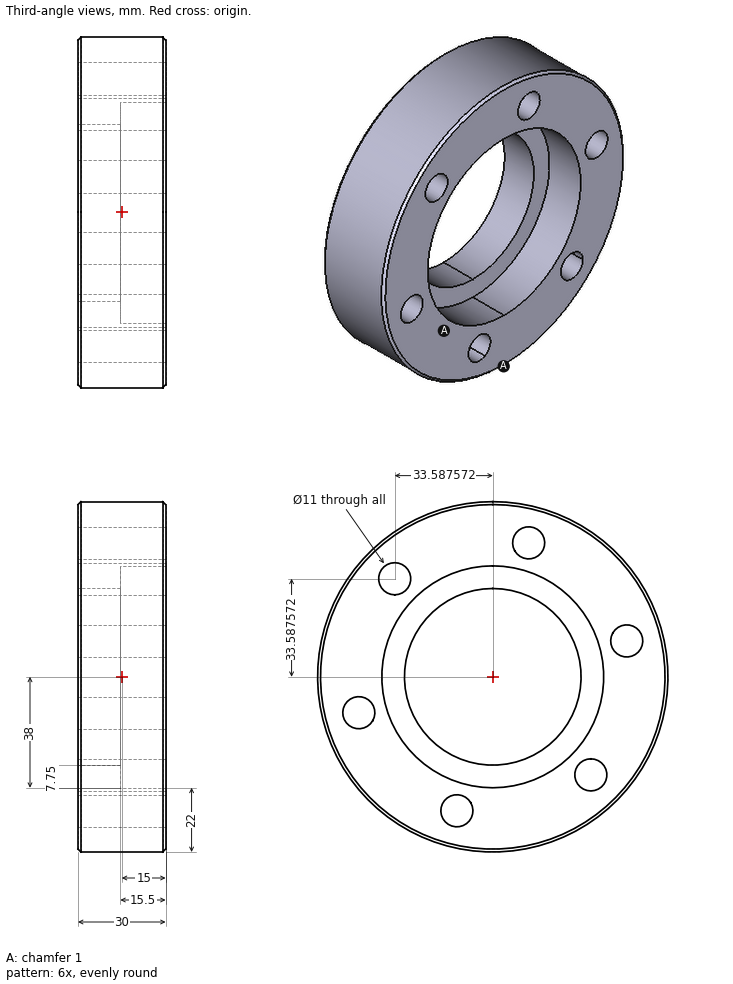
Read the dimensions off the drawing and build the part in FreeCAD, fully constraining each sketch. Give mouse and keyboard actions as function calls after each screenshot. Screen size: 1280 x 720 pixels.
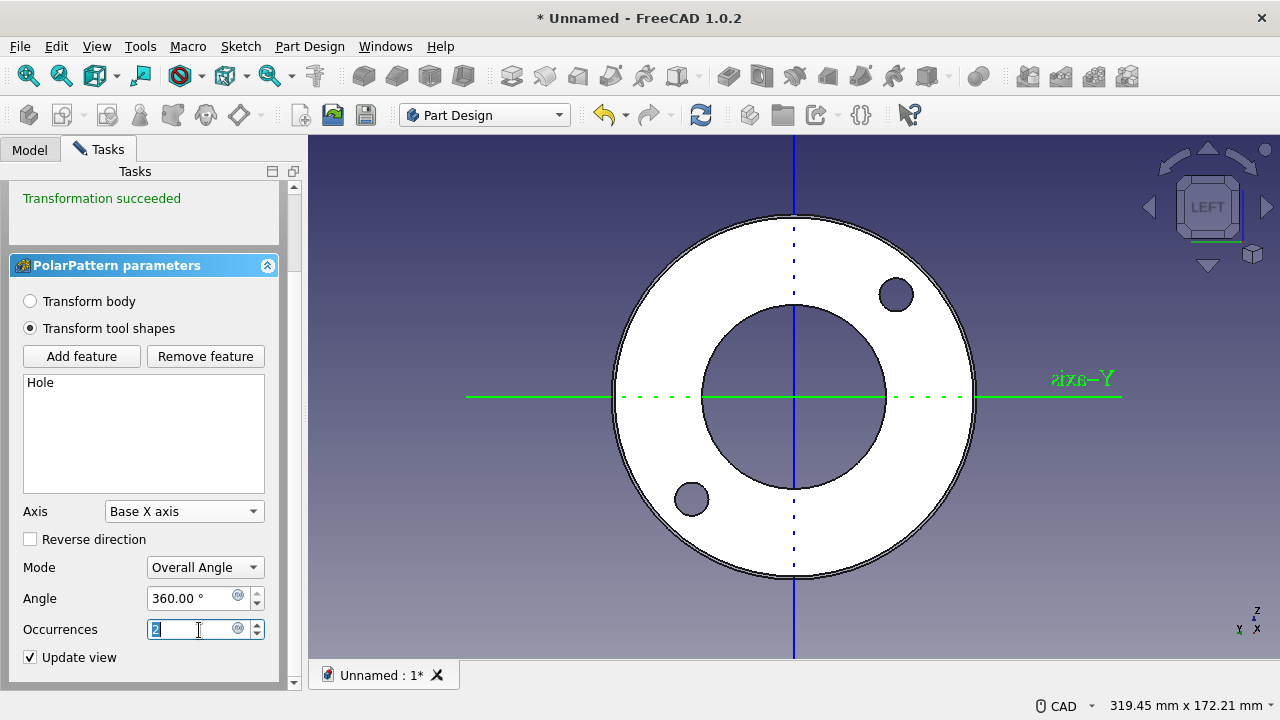
text(6)
key(Tab)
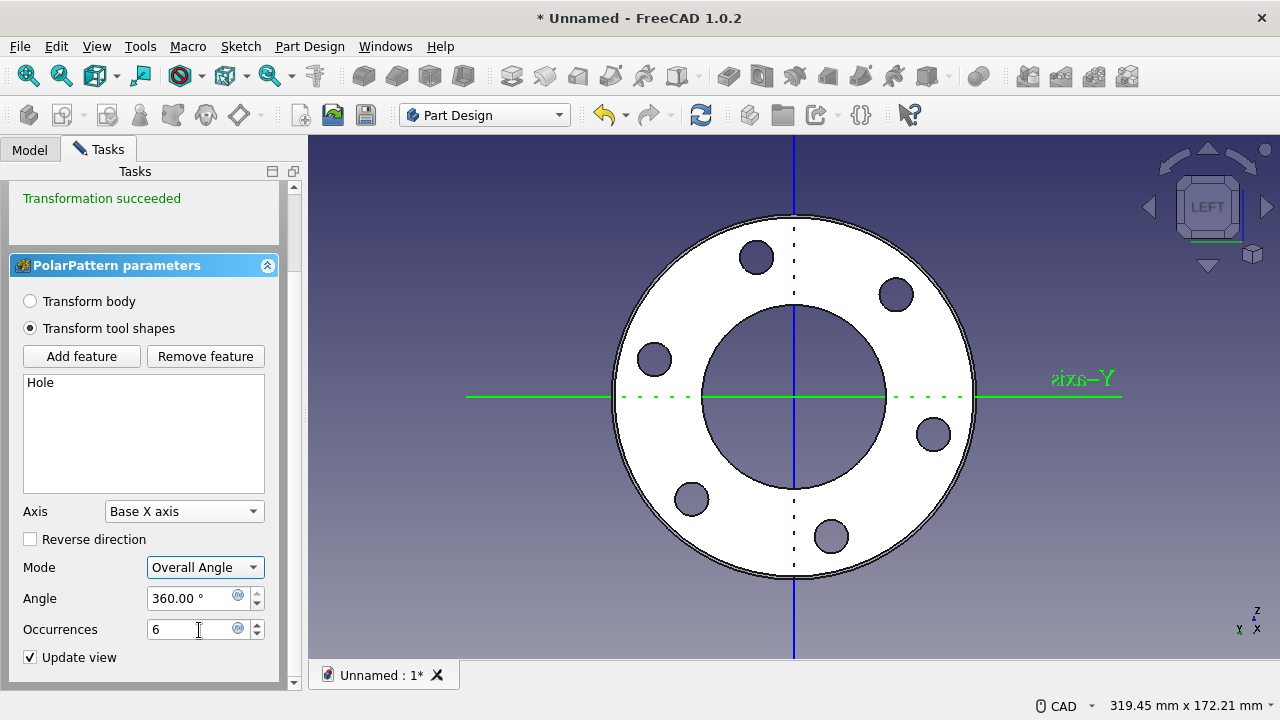
scroll(294, 436, up, 3)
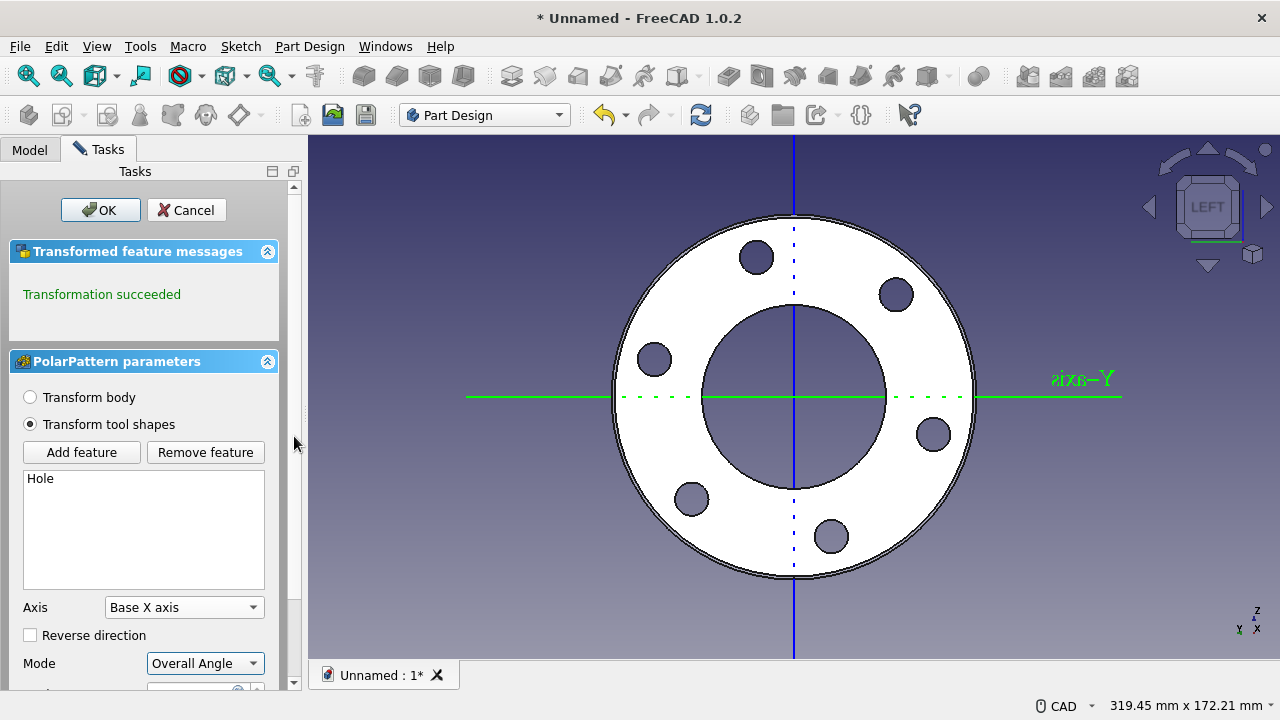
click(101, 210)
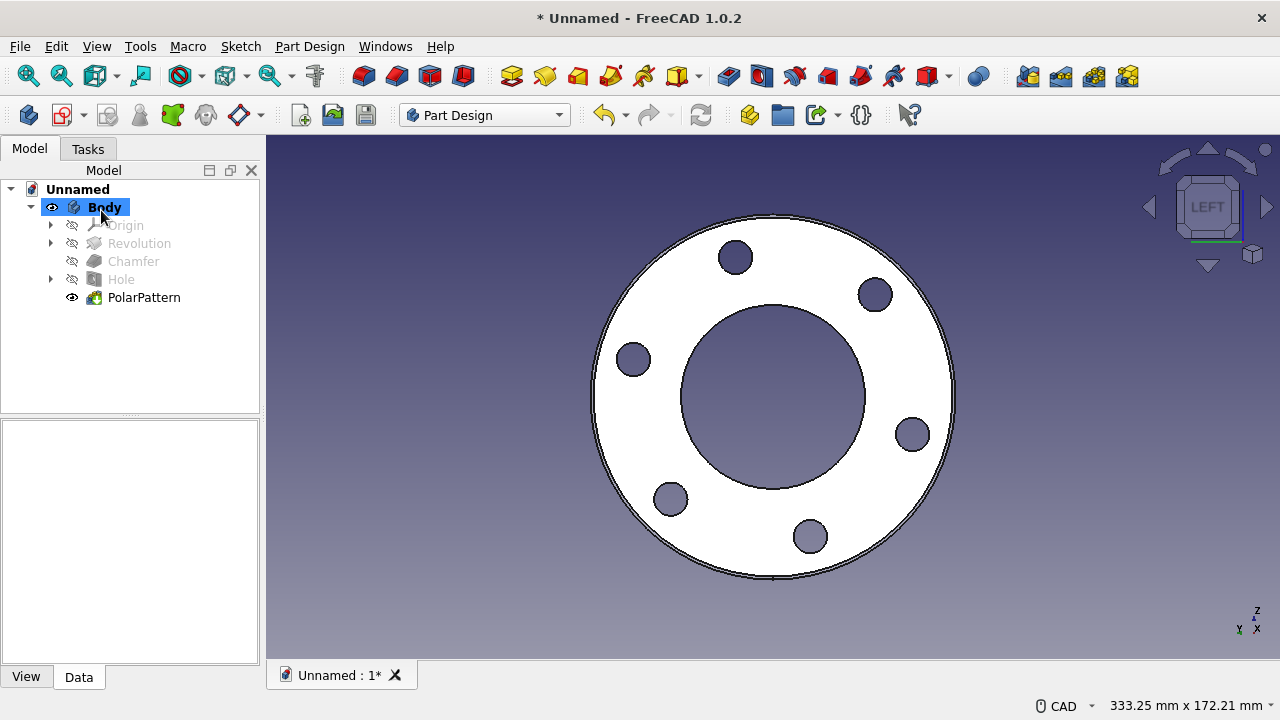
key(0)